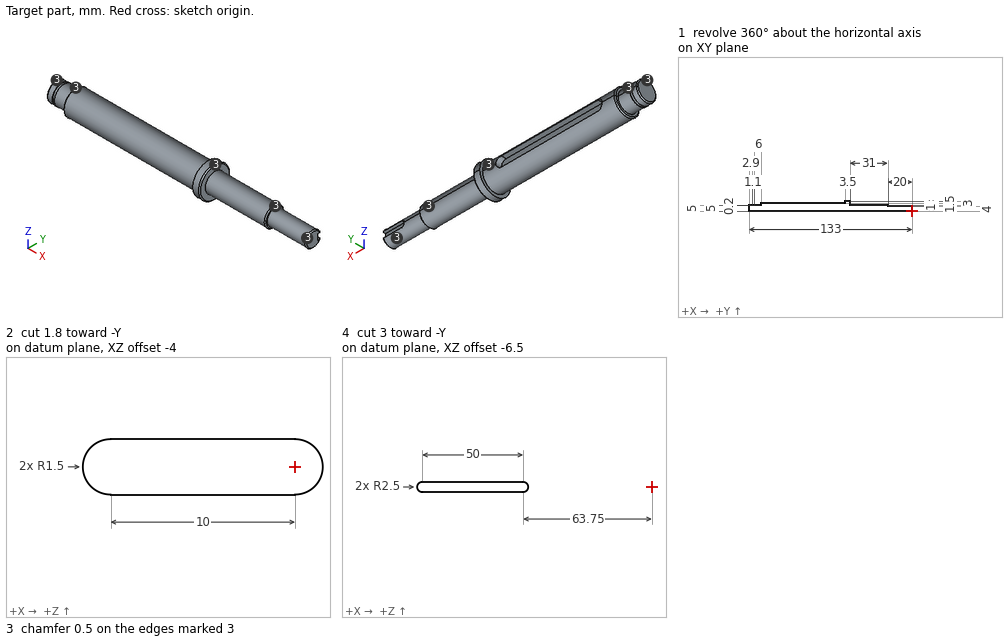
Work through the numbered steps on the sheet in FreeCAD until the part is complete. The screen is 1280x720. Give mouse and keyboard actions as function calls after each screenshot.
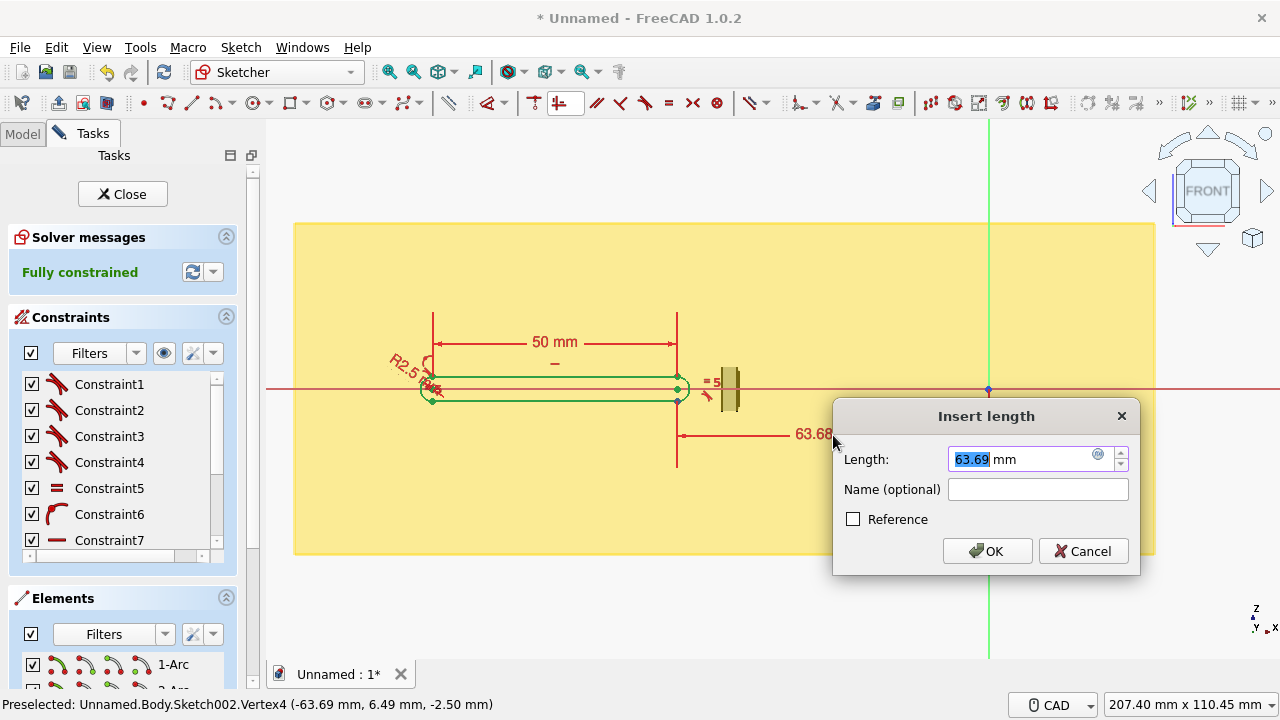
text(63.75)
key(Return)
key(Escape)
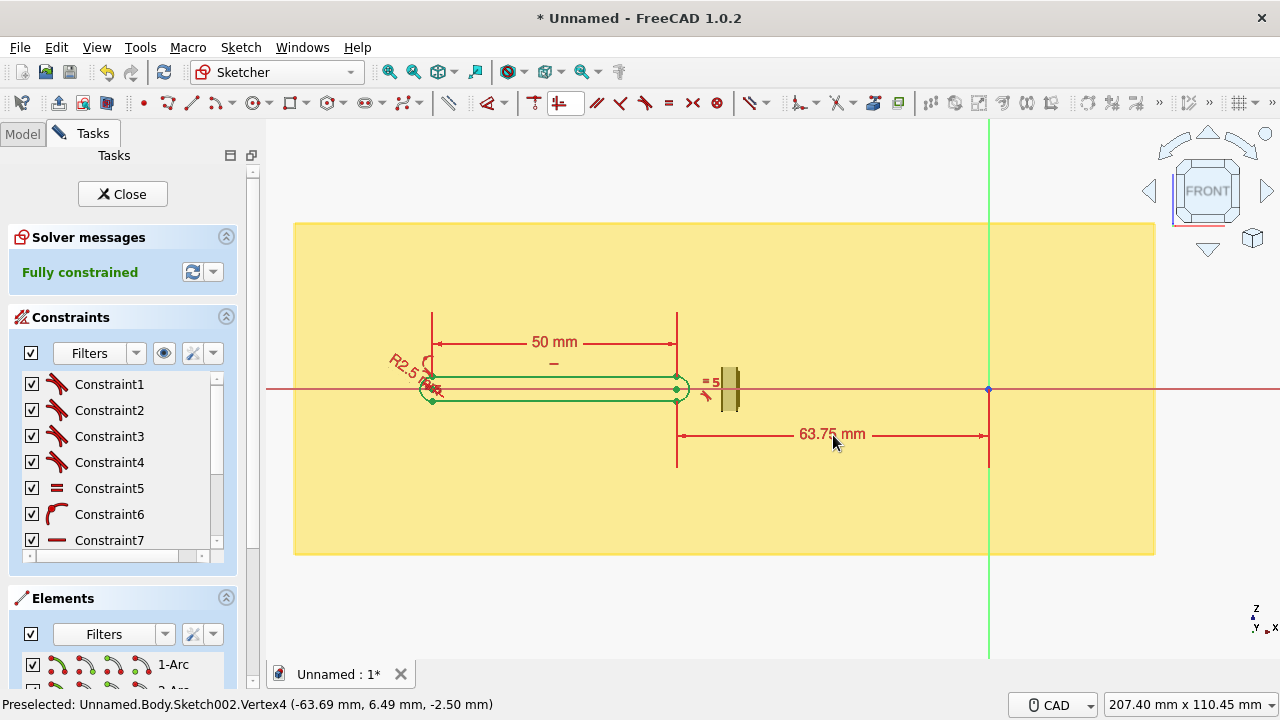
click(123, 194)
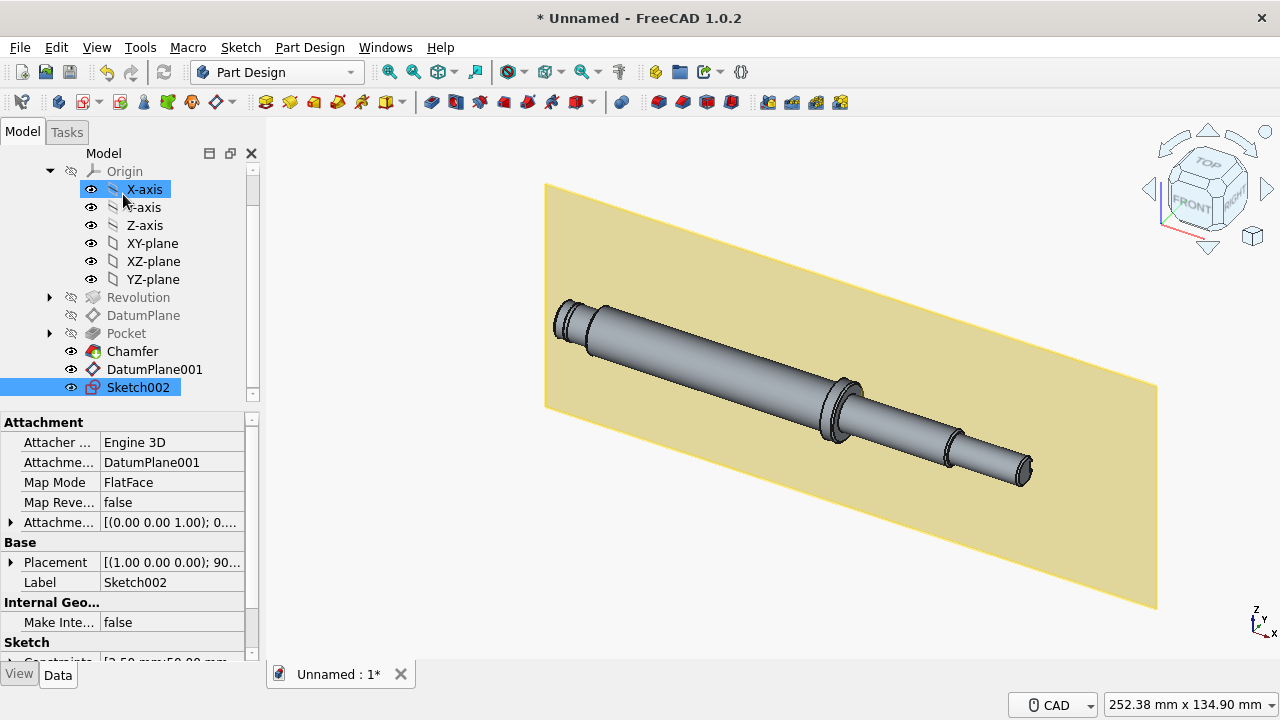
click(432, 102)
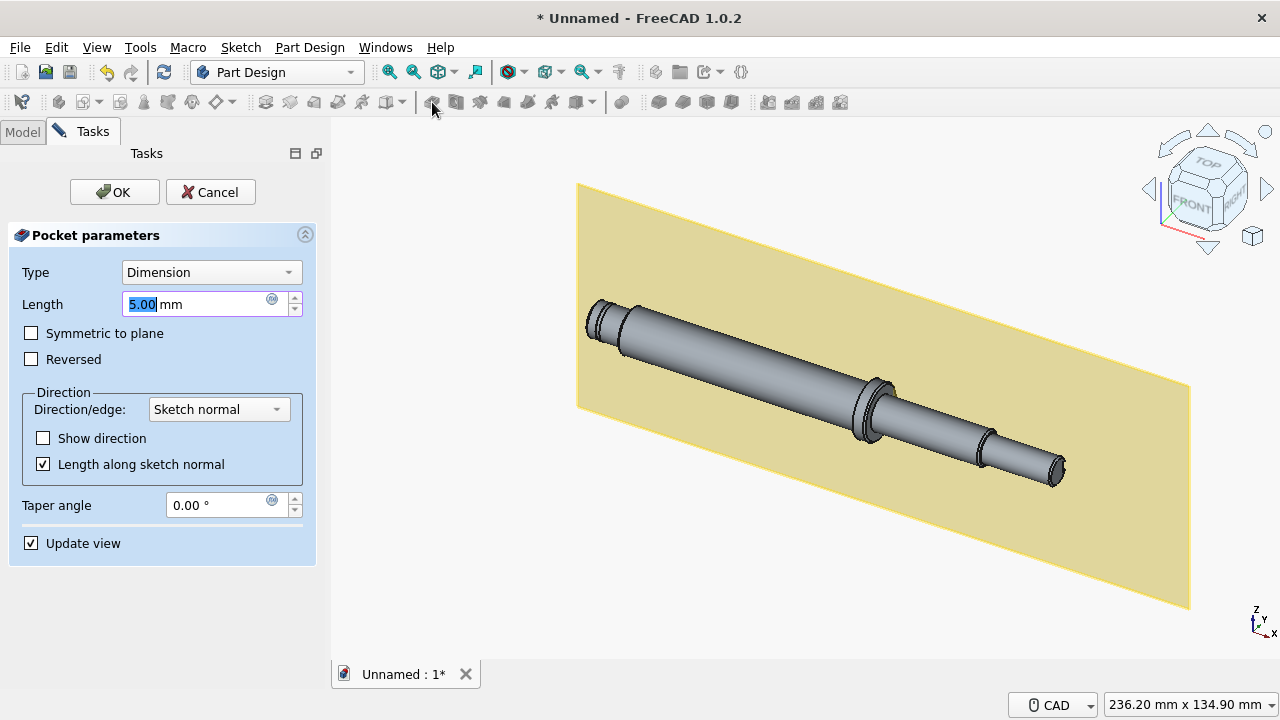
text(3)
key(Tab)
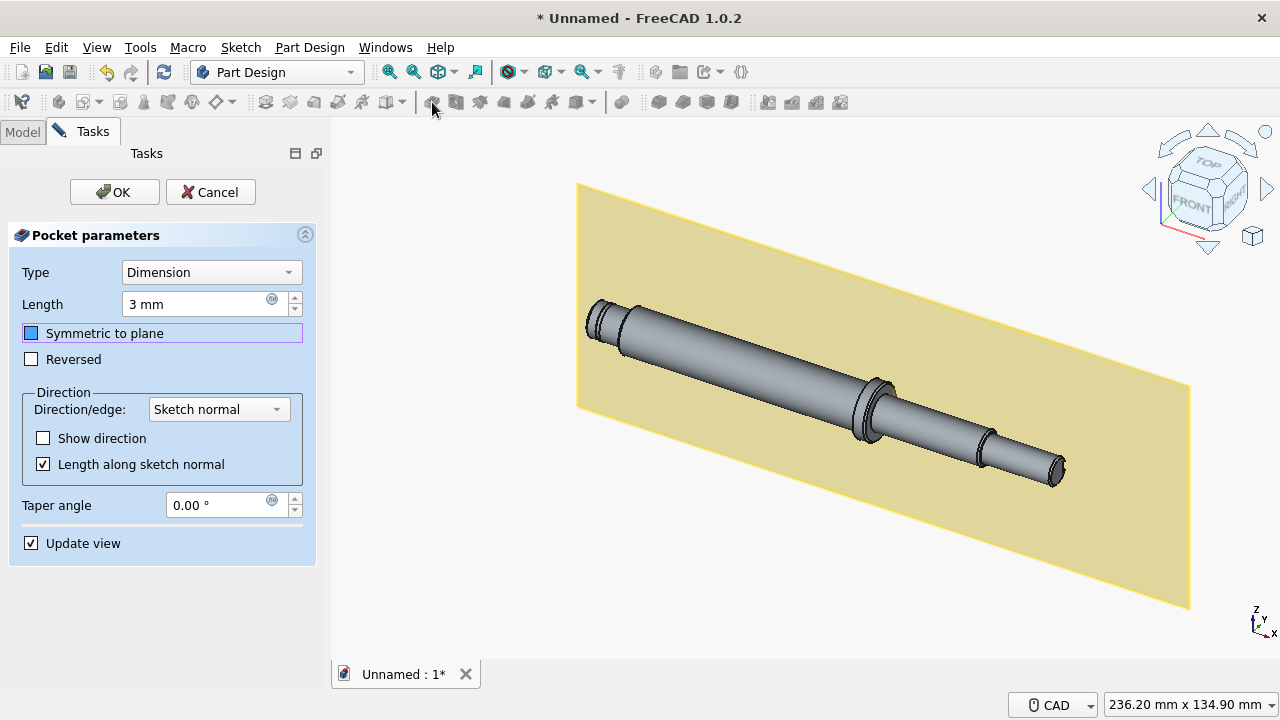
click(30, 359)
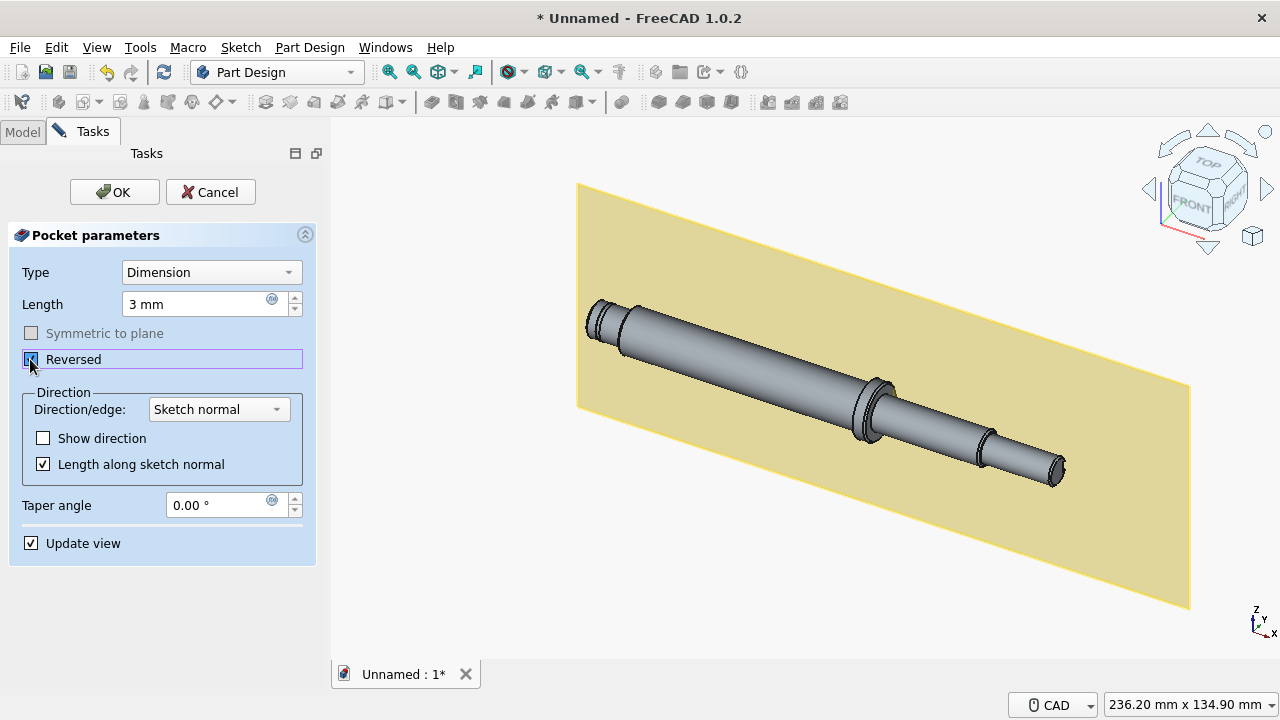
click(115, 192)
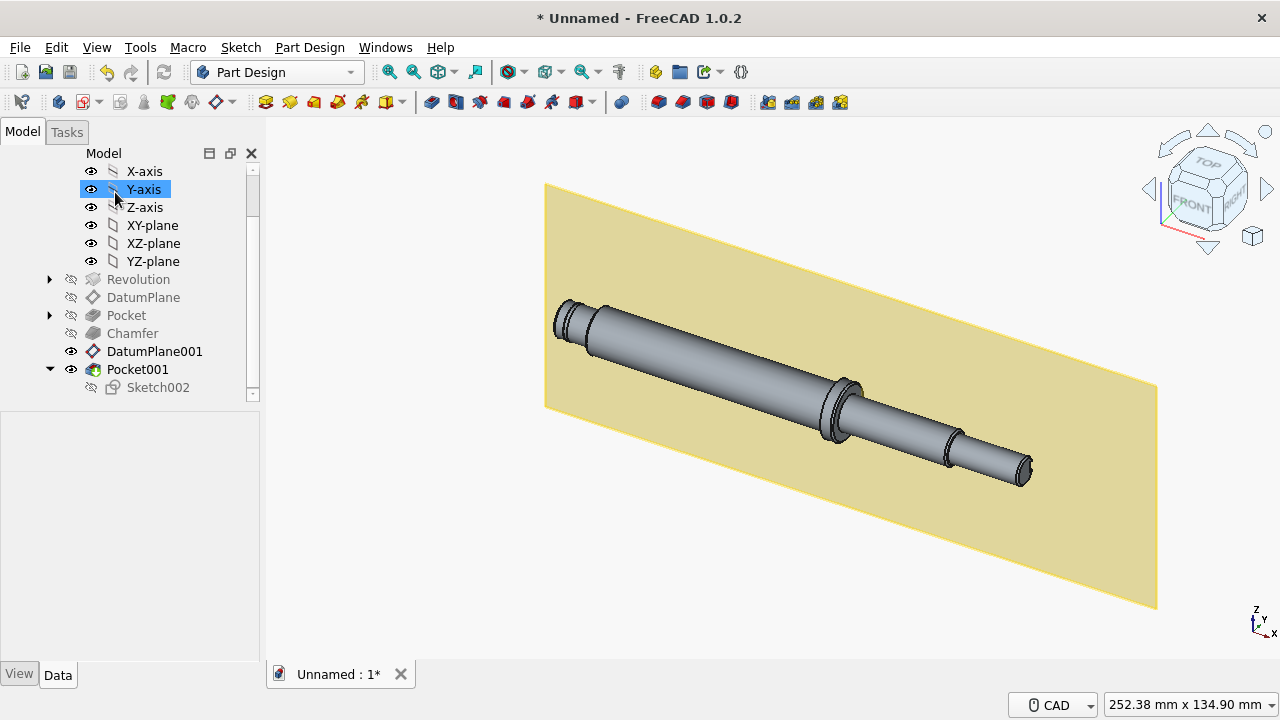
click(116, 351)
key(space)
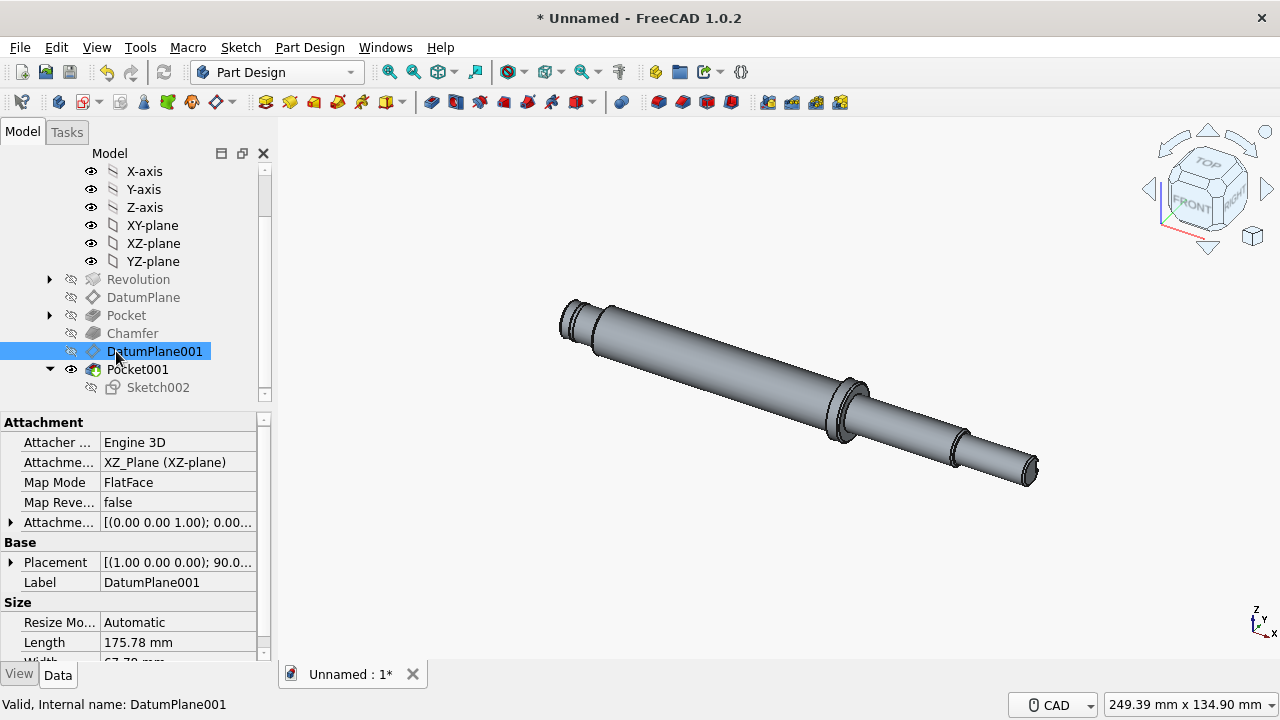
key(0)